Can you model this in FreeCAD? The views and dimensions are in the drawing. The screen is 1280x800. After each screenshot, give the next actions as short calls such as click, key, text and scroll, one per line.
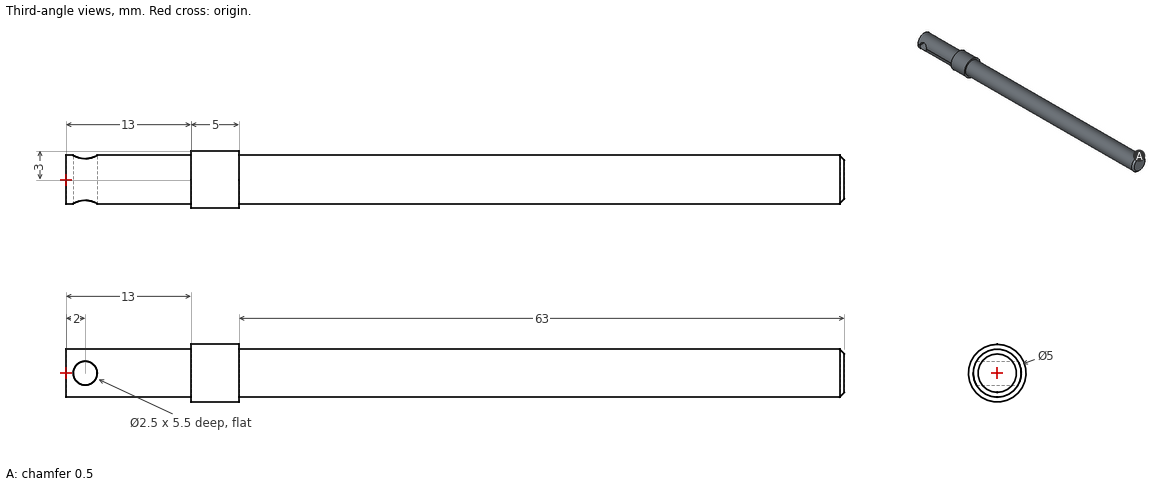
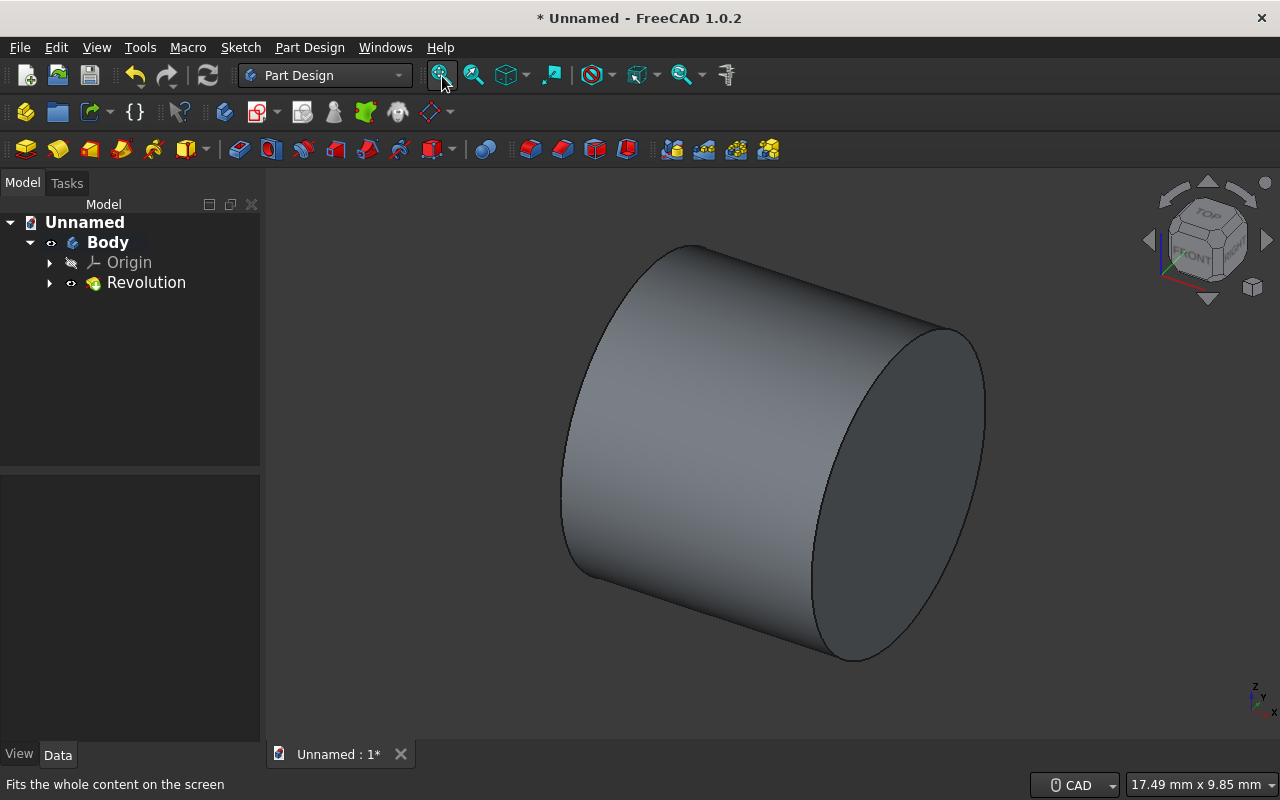
key(6)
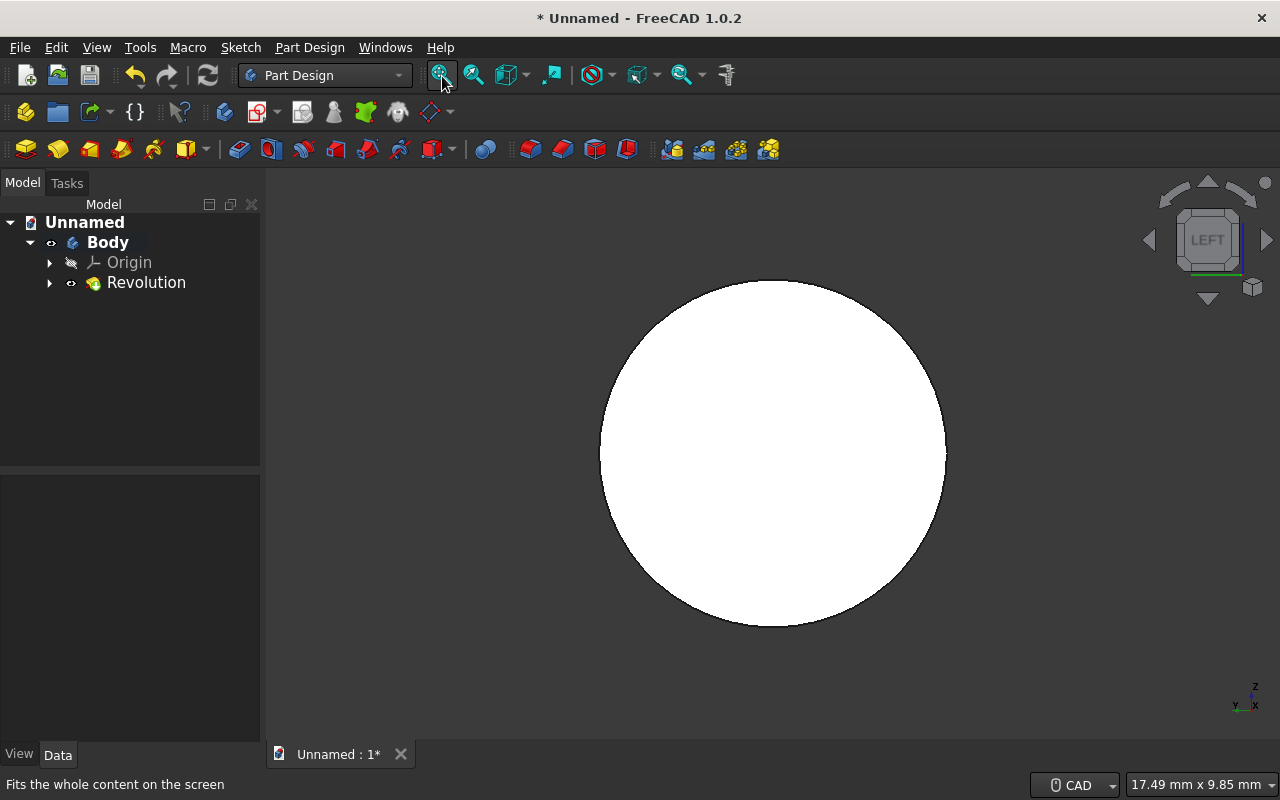
click(773, 452)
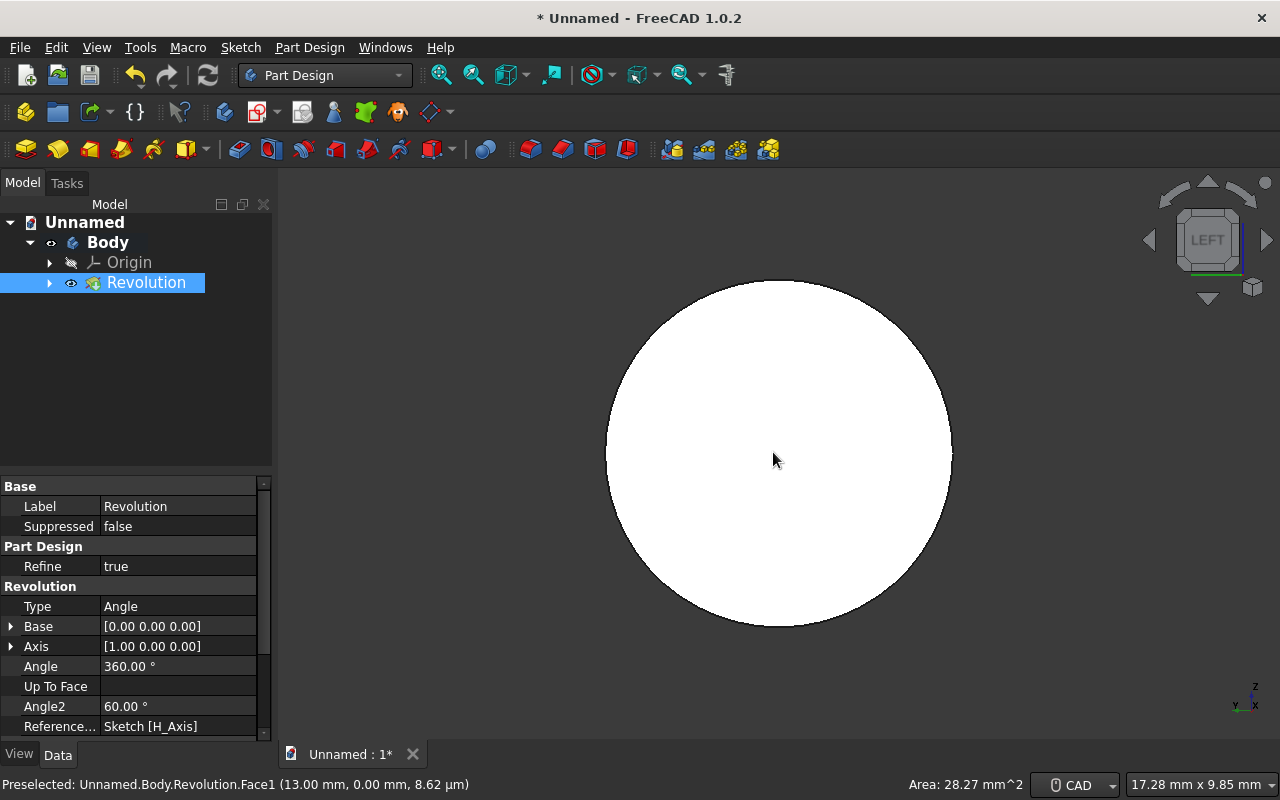
click(258, 112)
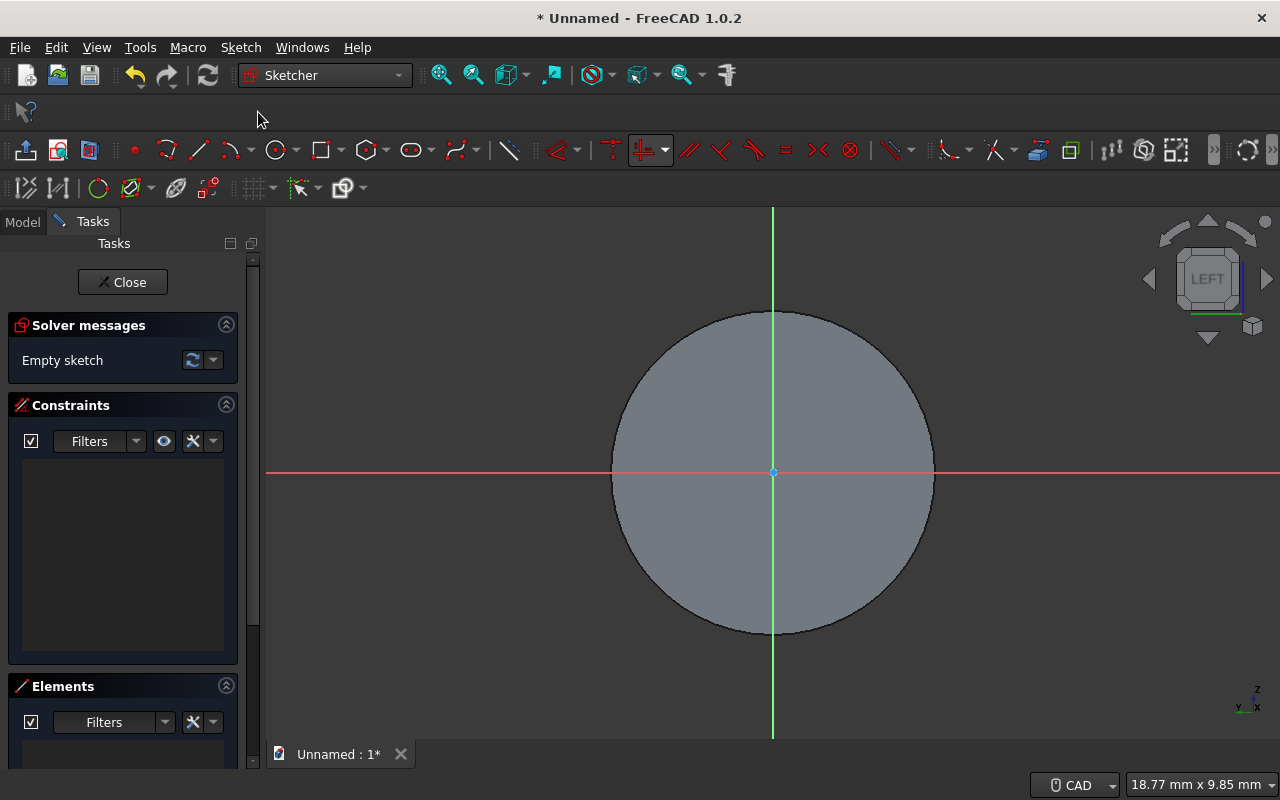
click(276, 150)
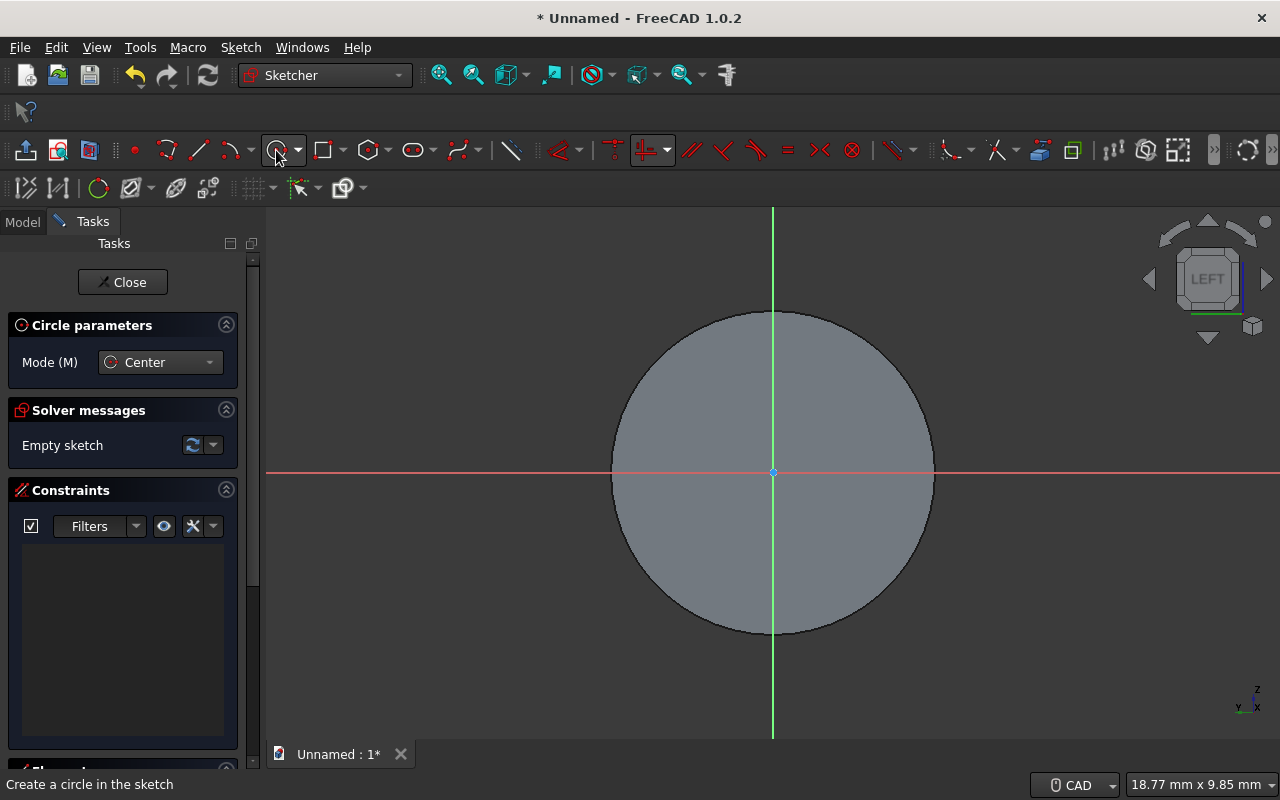
click(773, 473)
move(868, 378)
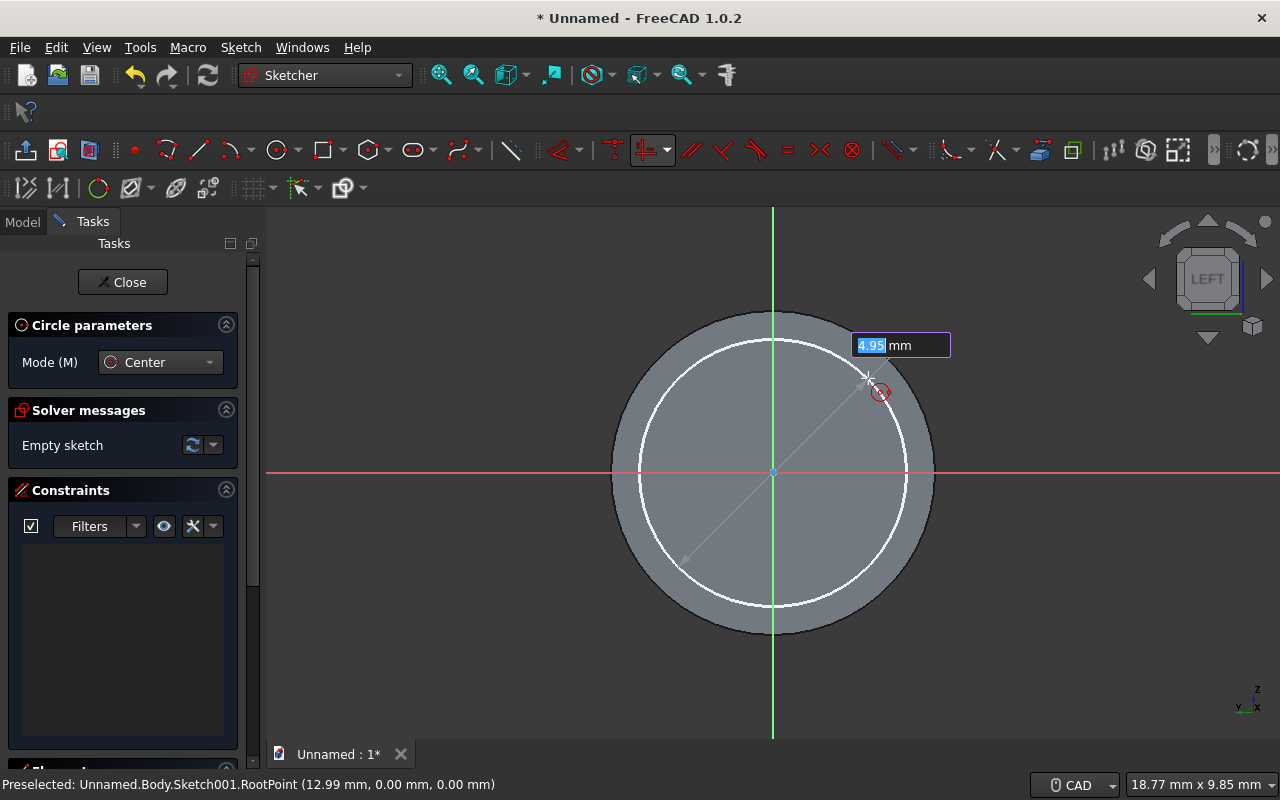
text(5)
key(Return)
key(Escape)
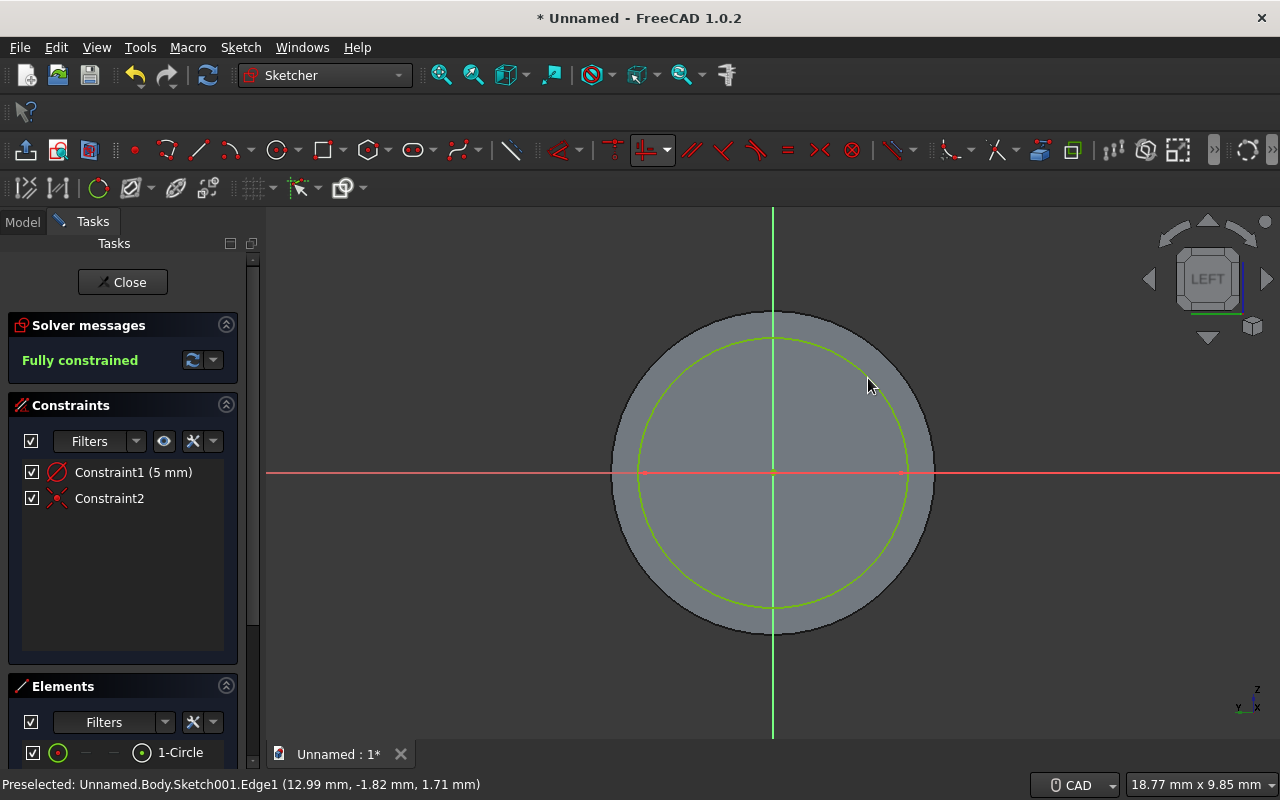
click(123, 282)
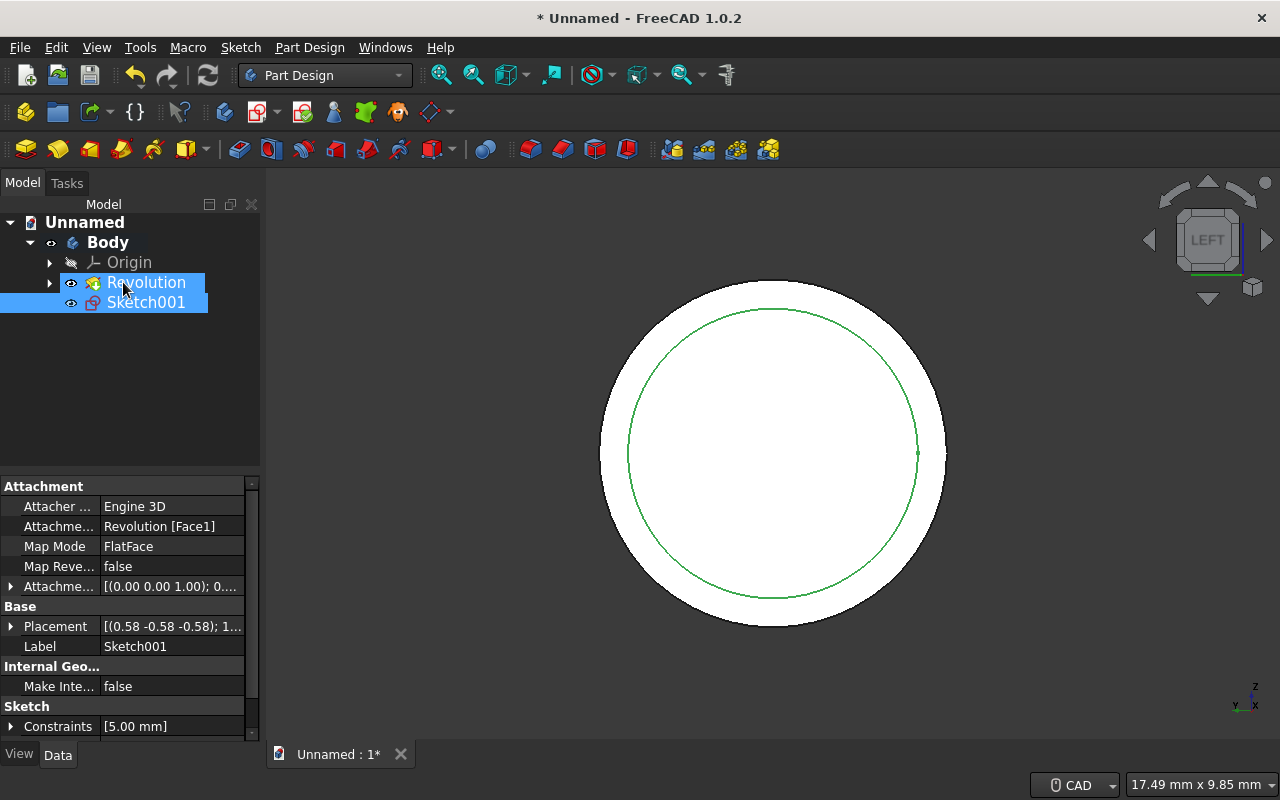
click(26, 150)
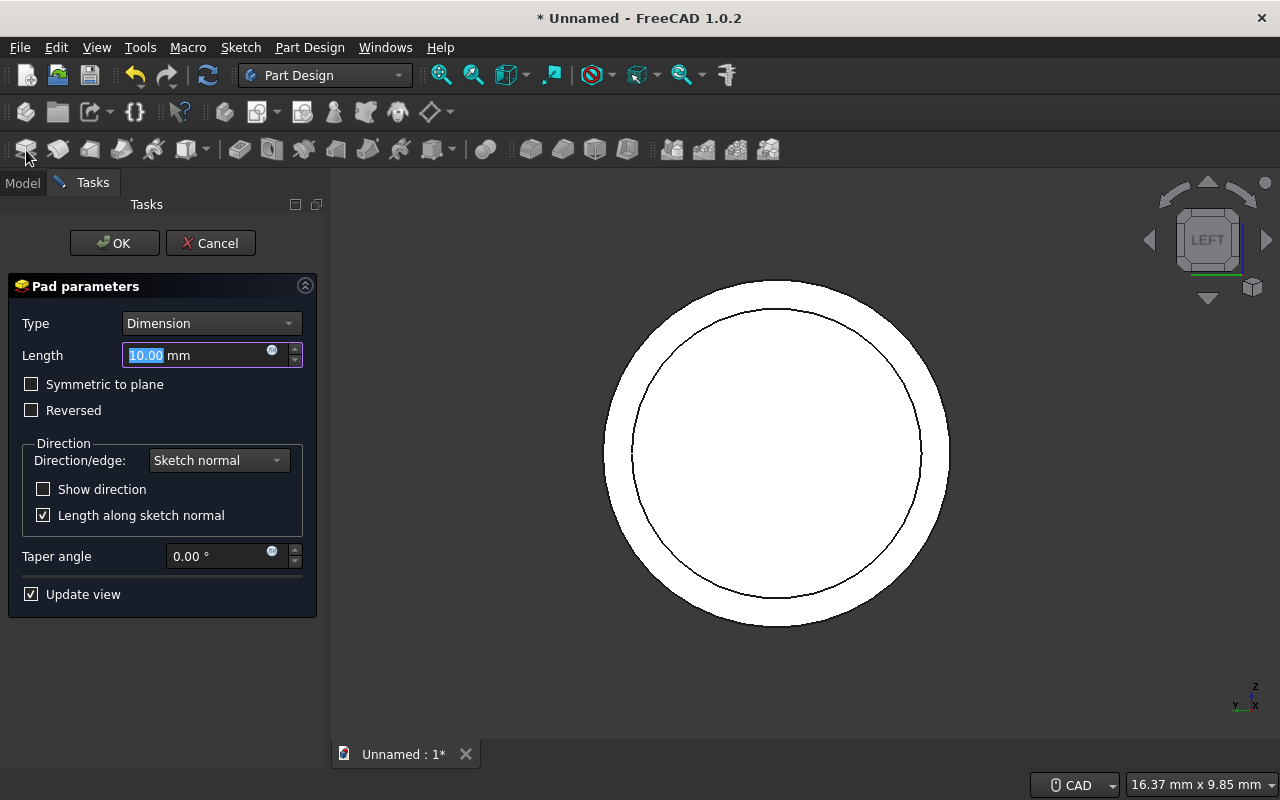
text(13)
key(Tab)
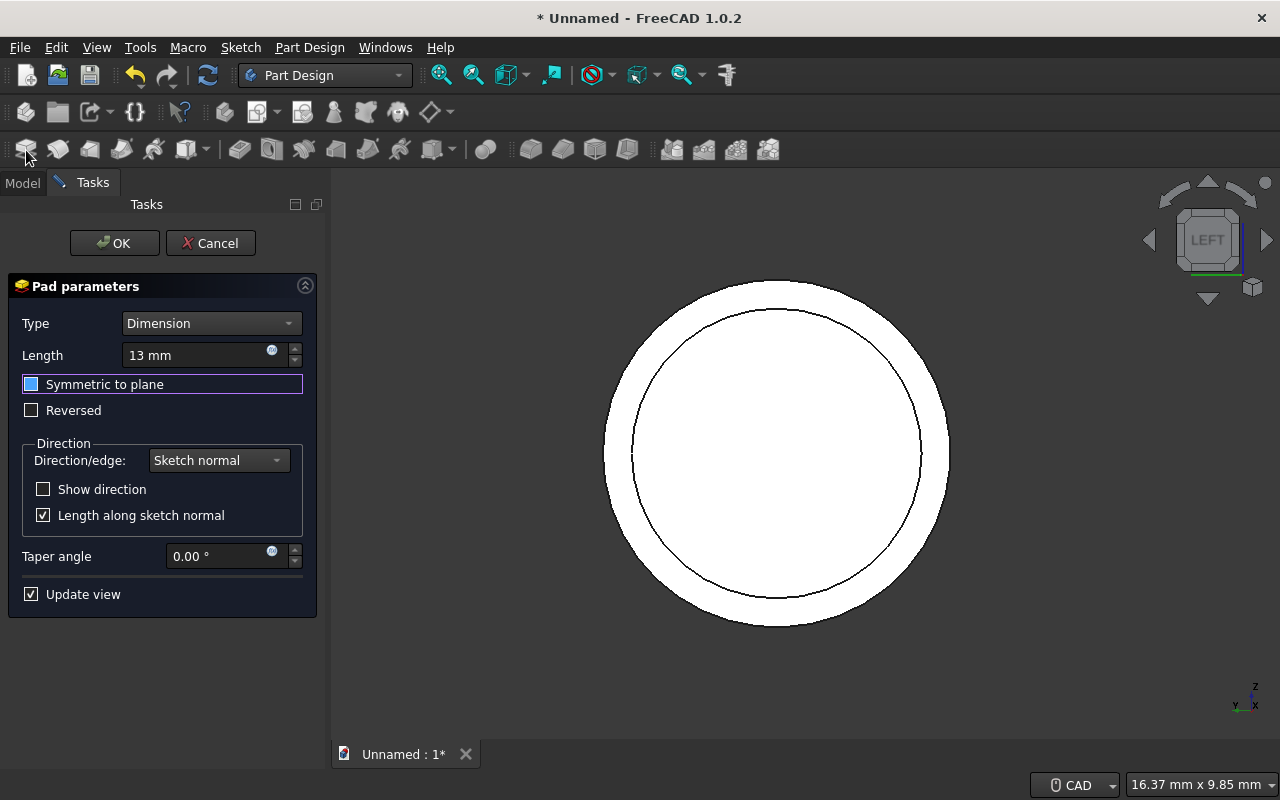
click(115, 243)